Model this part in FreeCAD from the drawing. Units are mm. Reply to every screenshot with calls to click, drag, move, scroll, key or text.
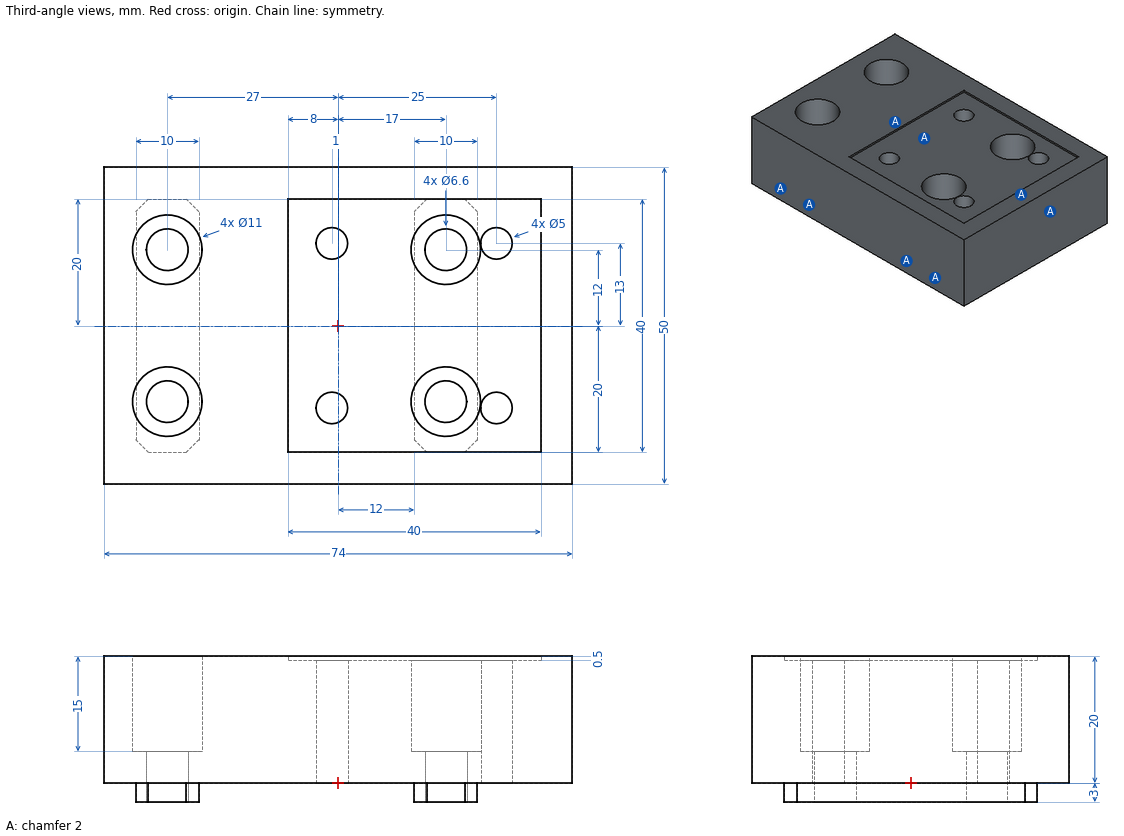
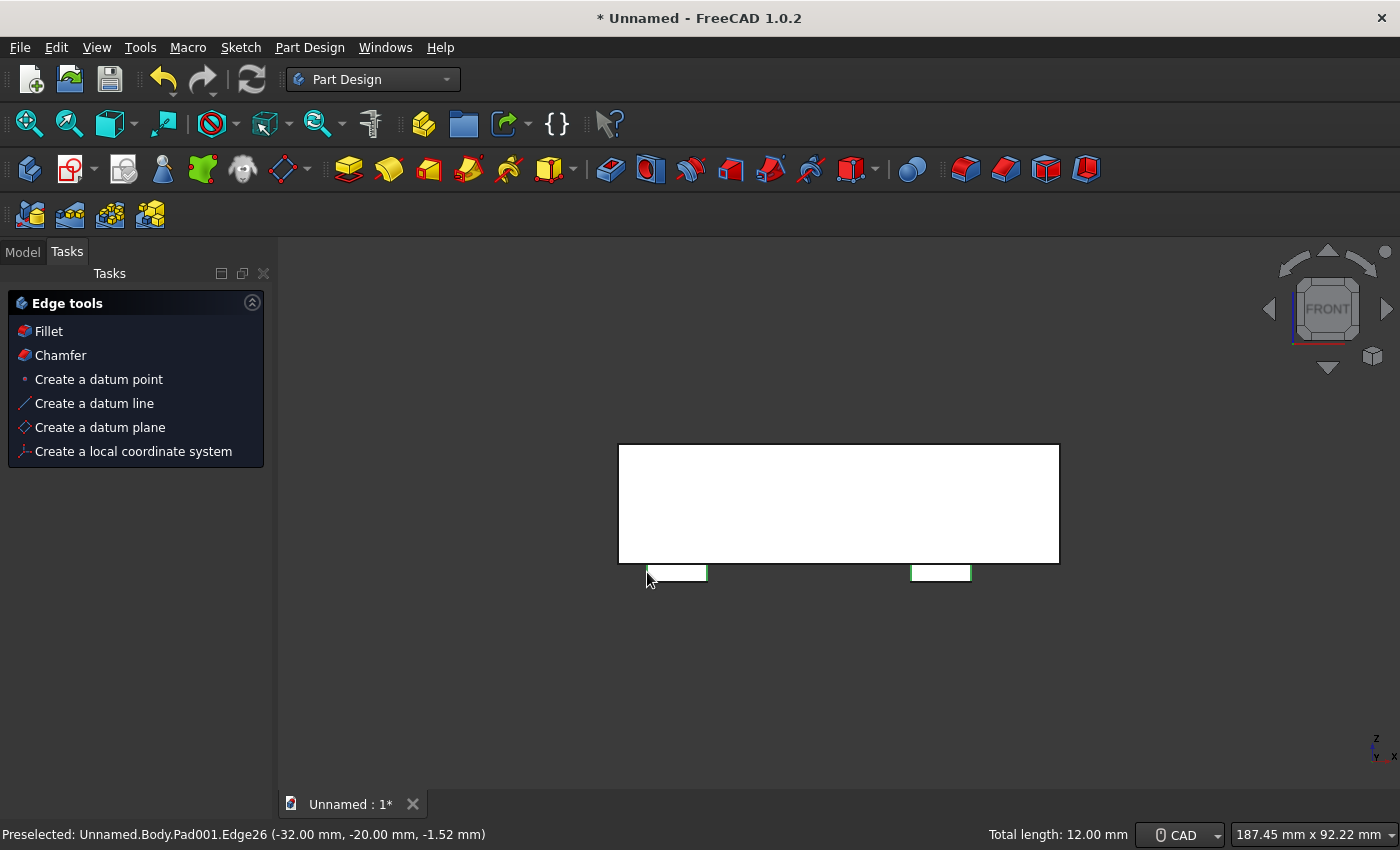
scroll(971, 572, up, 5)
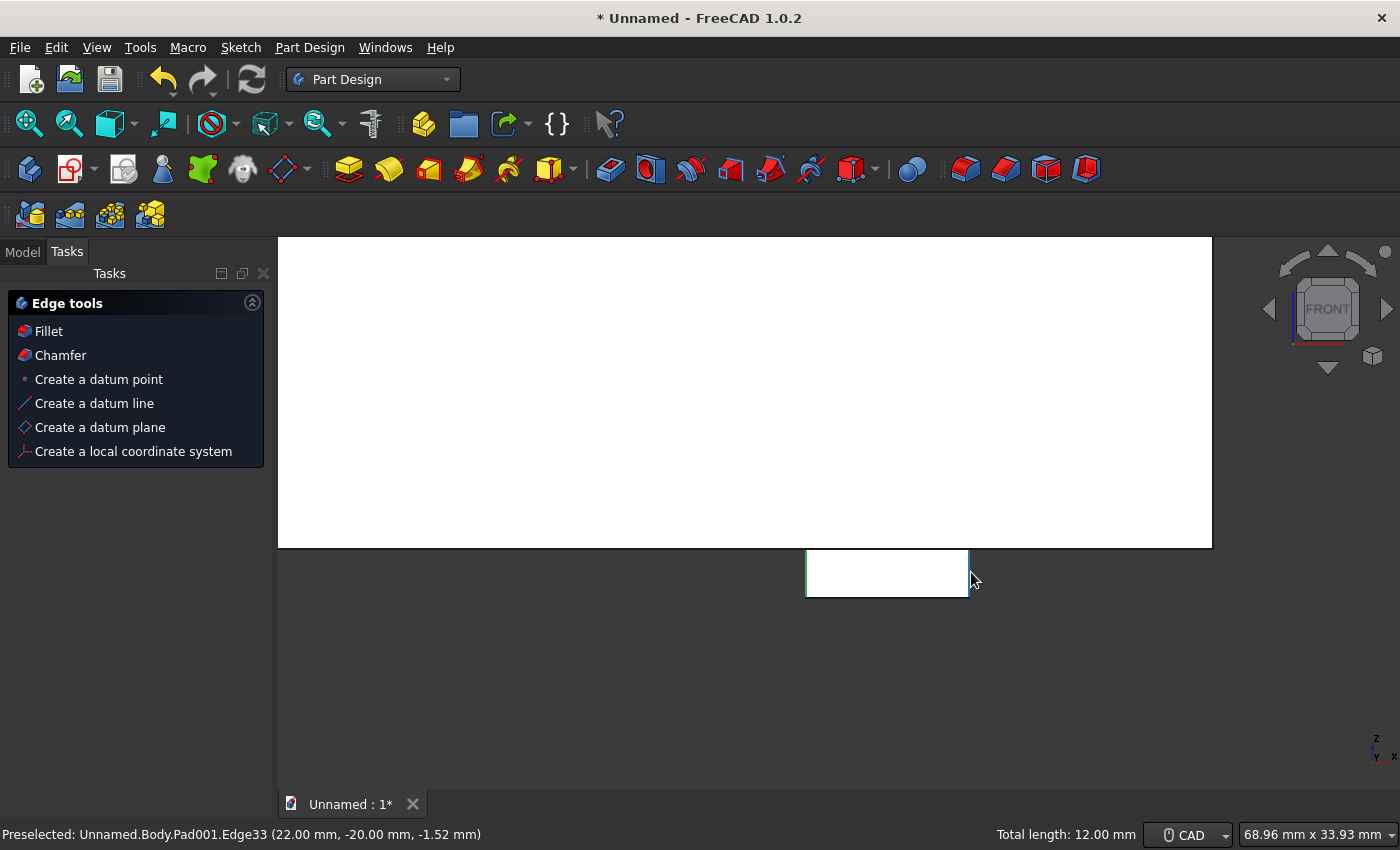
click(30, 124)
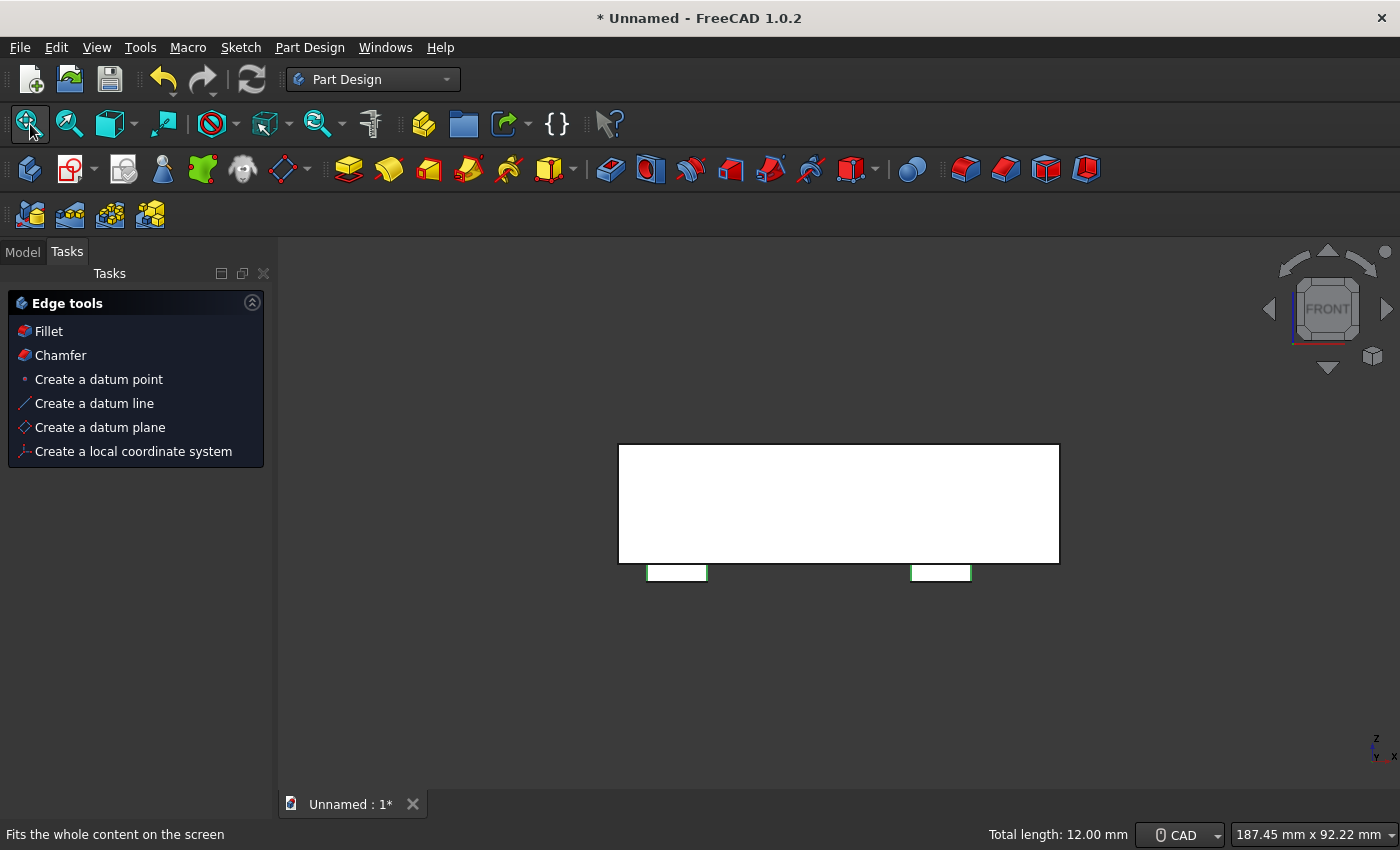
key(3)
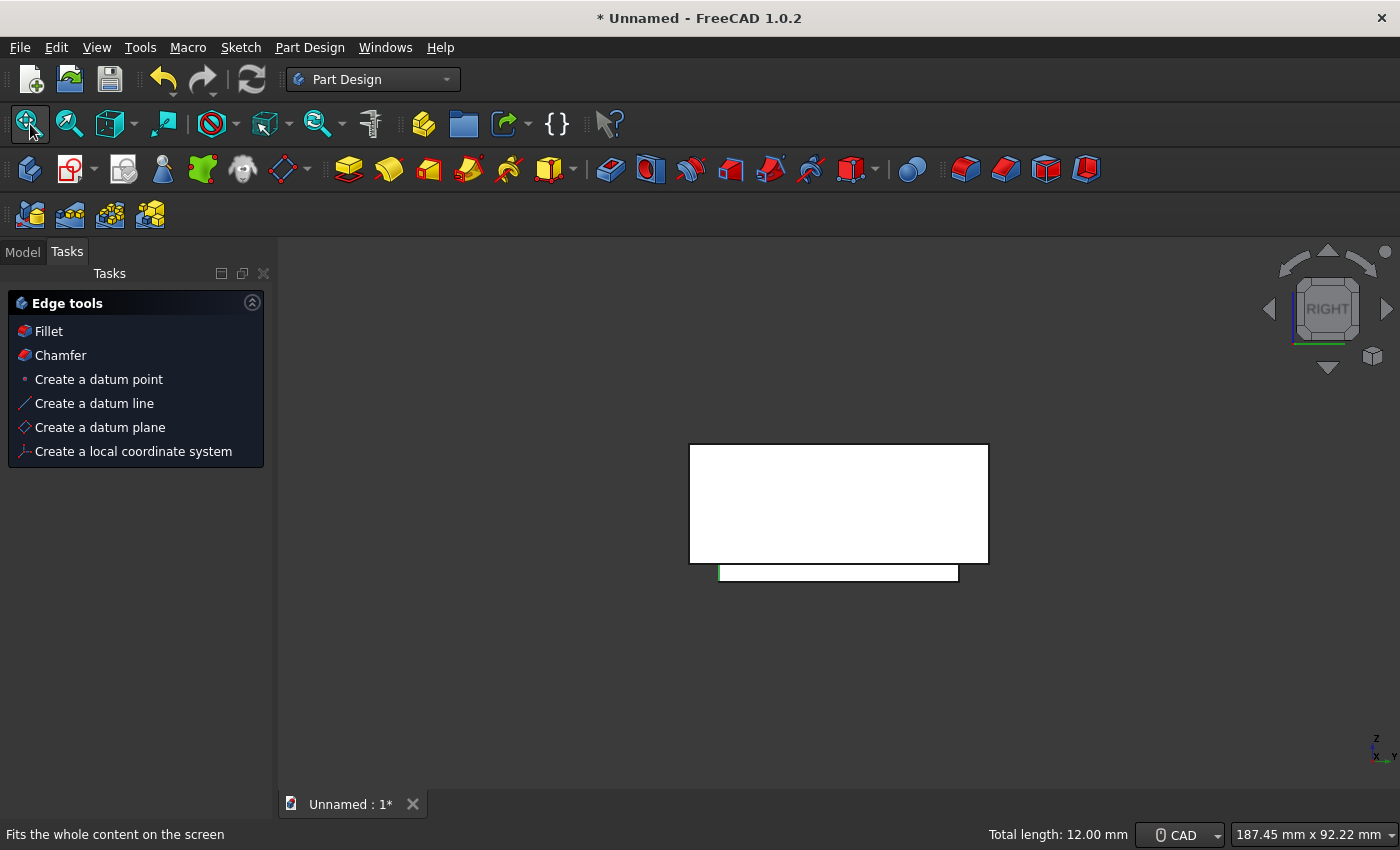
click(30, 124)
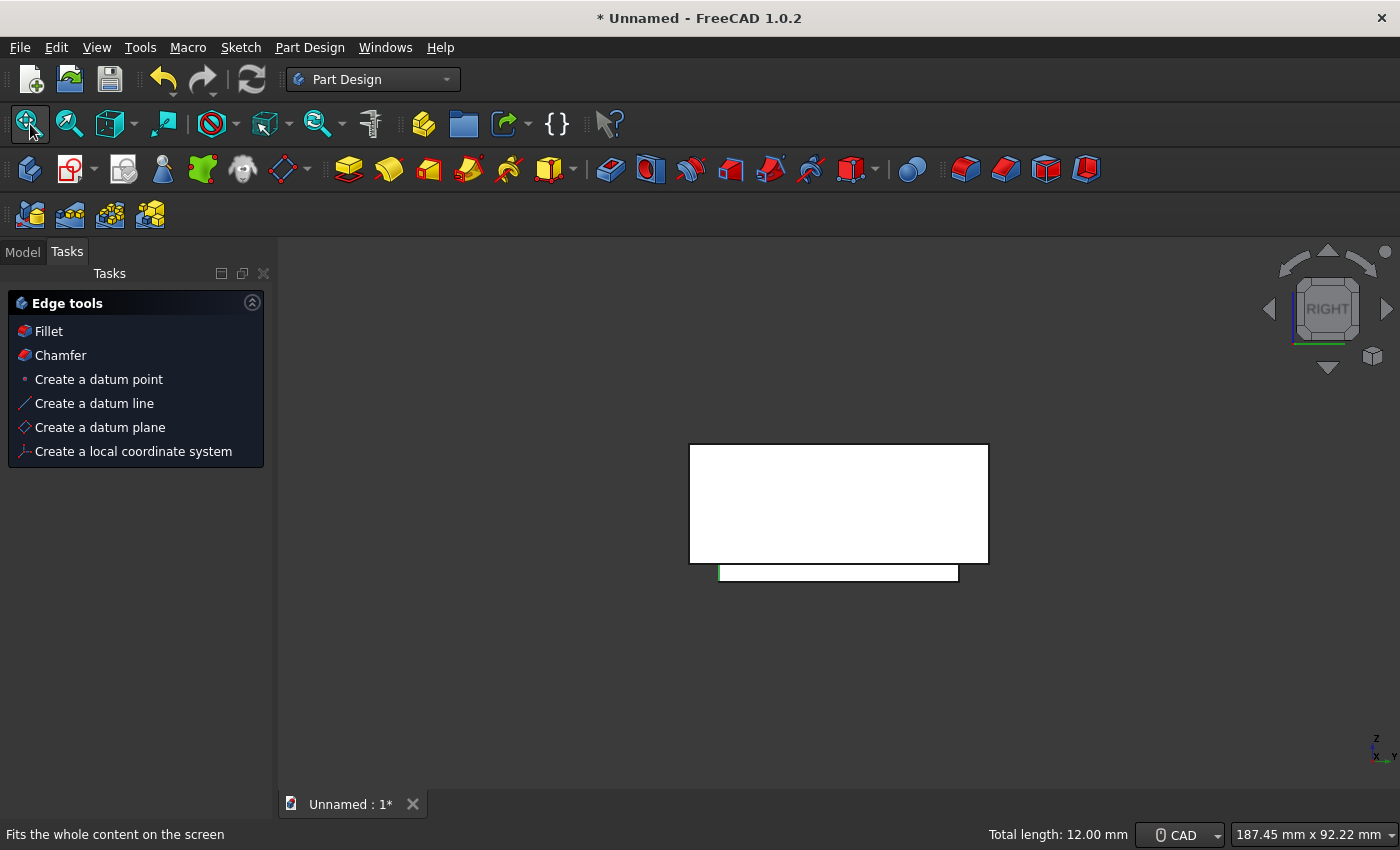
click(959, 572, ctrl)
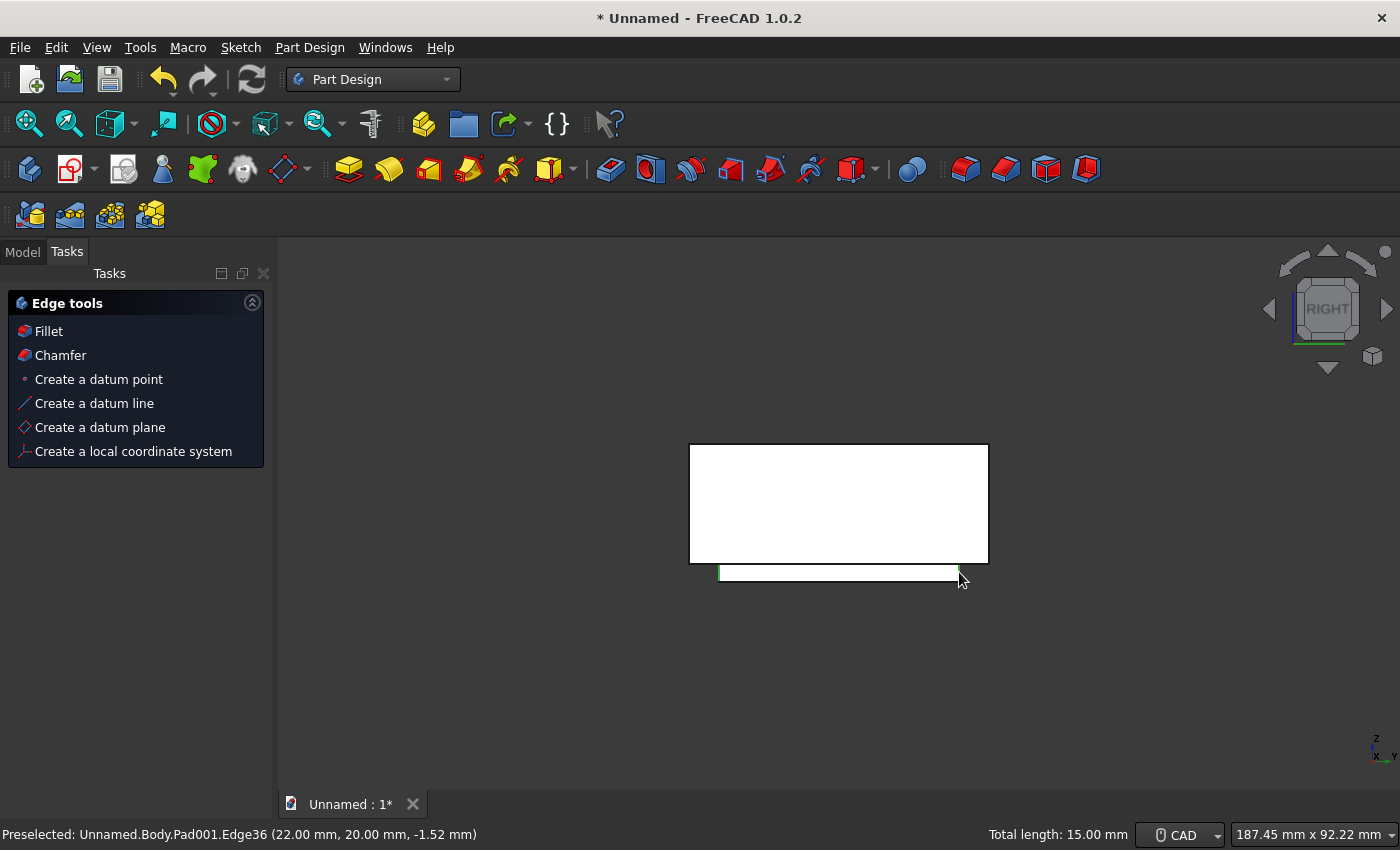
scroll(959, 572, up, 5)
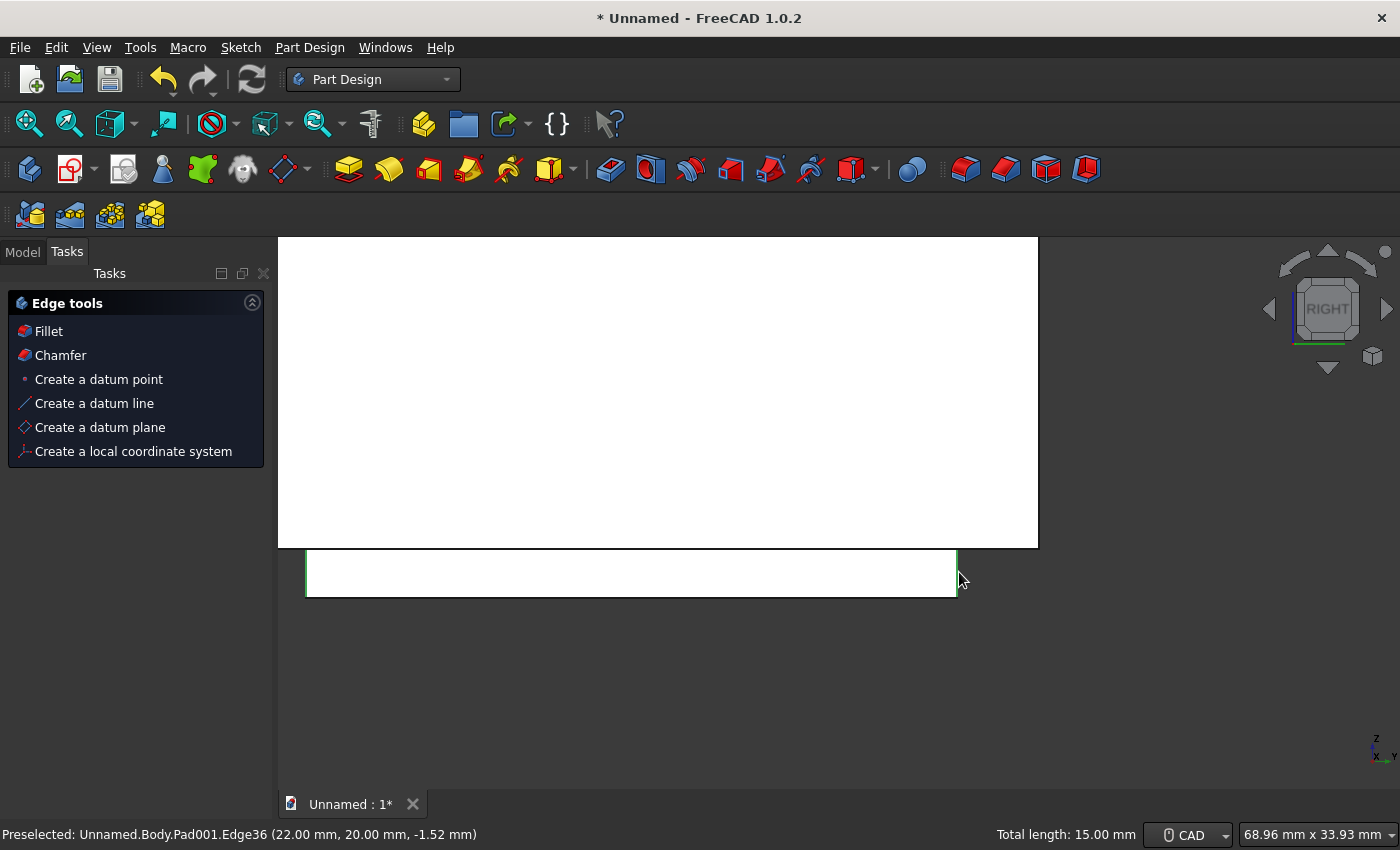
click(30, 124)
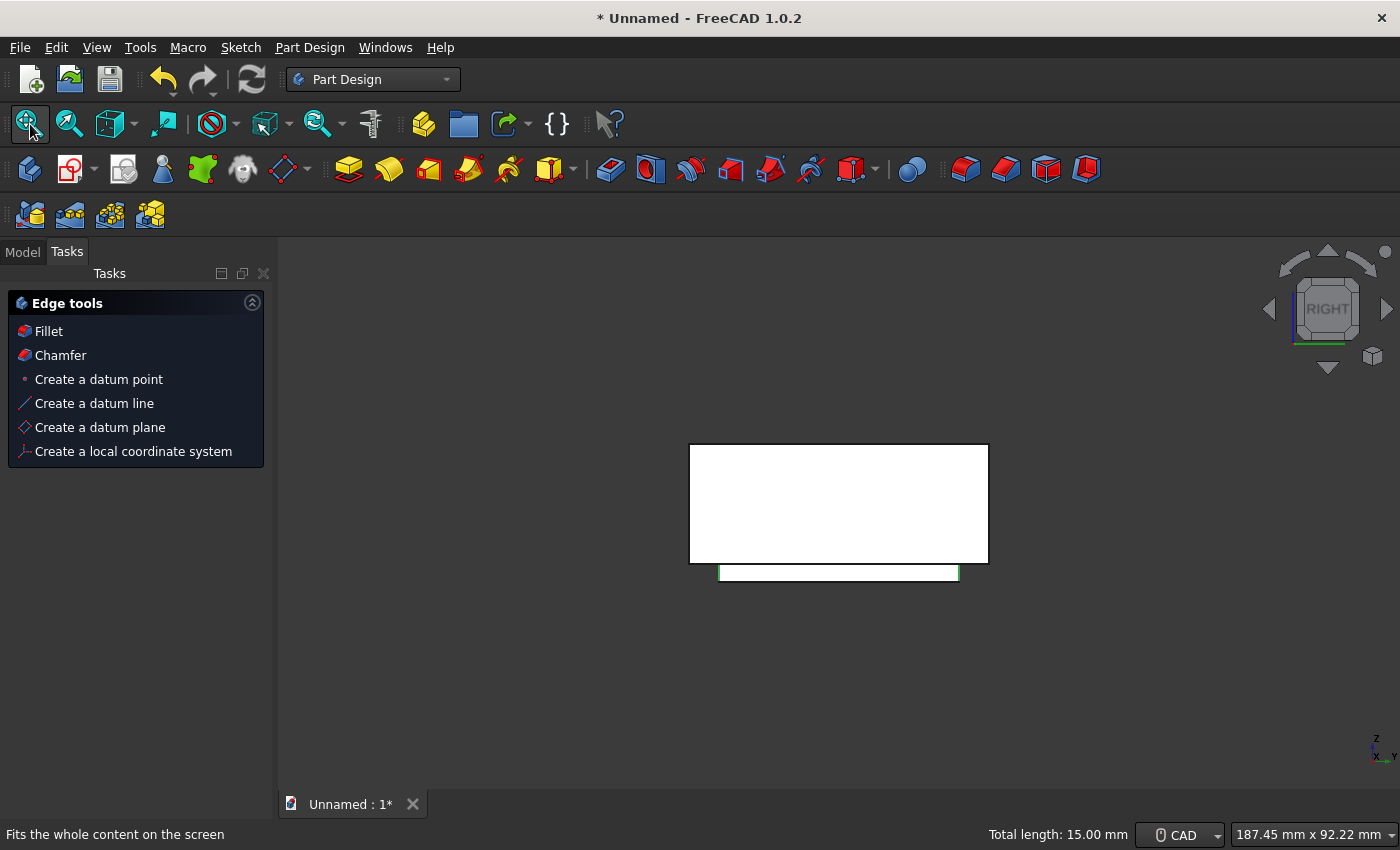
key(5)